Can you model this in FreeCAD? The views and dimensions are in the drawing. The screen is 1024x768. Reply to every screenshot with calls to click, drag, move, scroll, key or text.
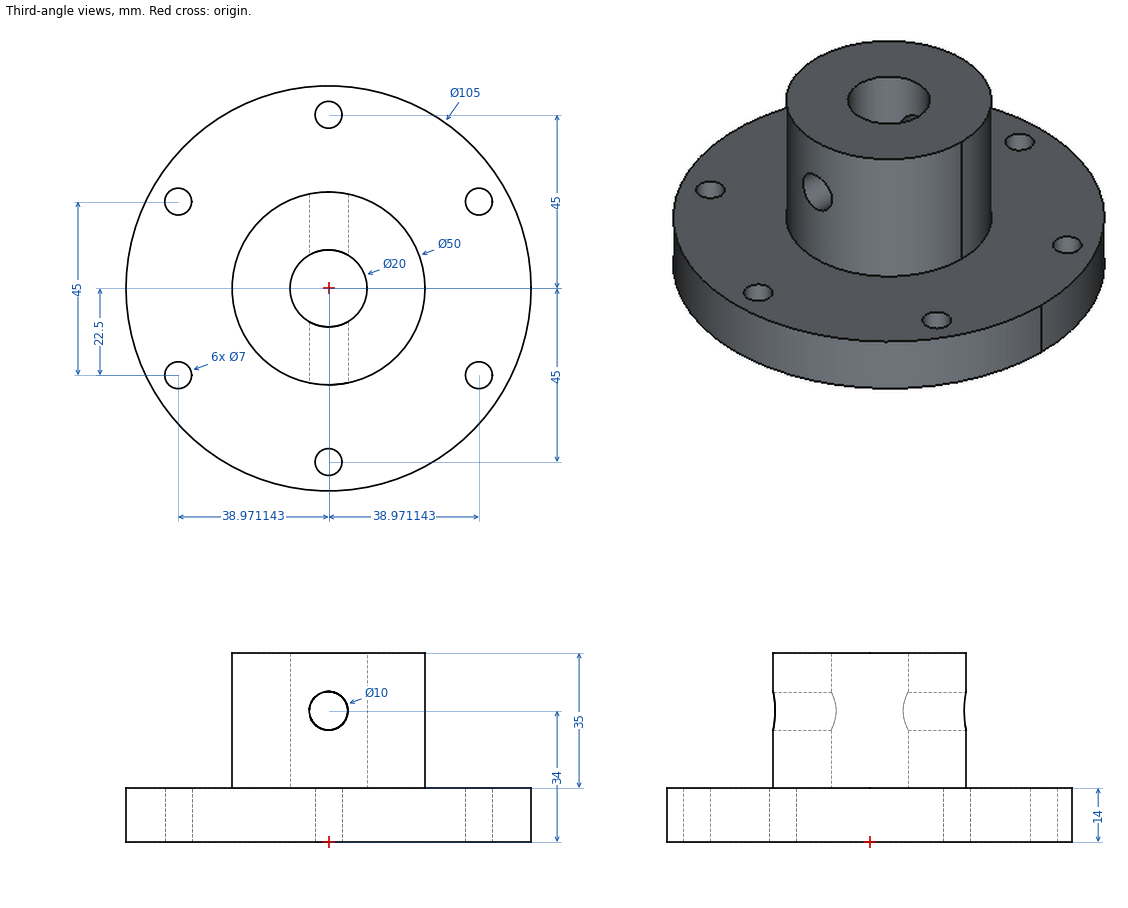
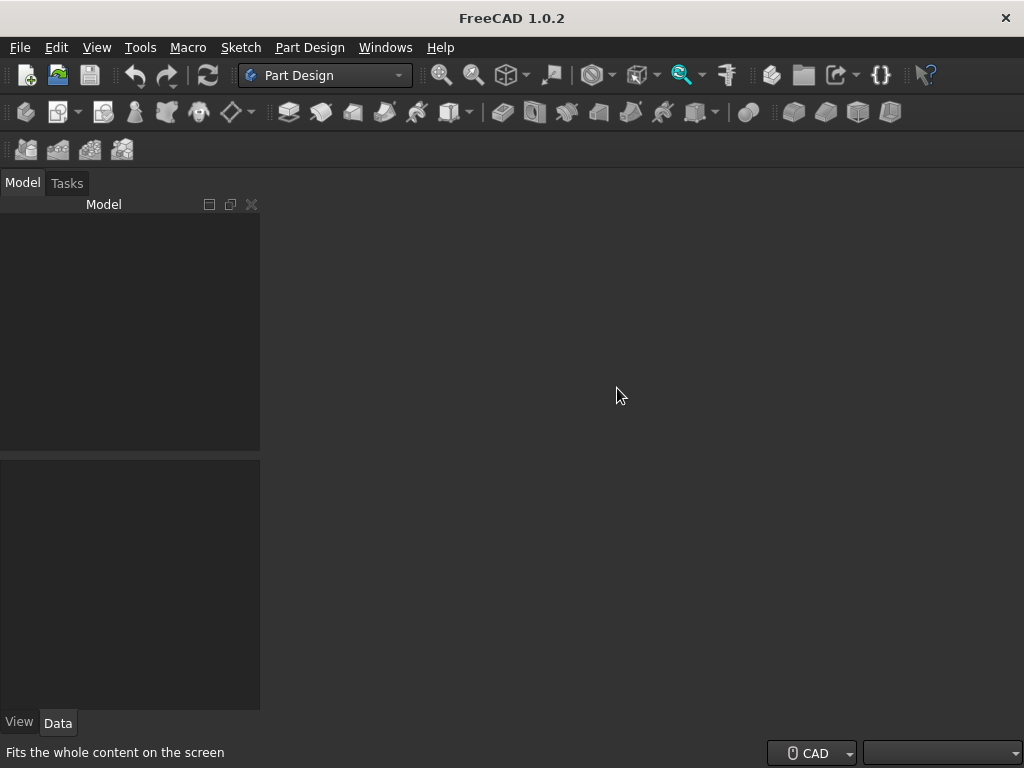
click(26, 76)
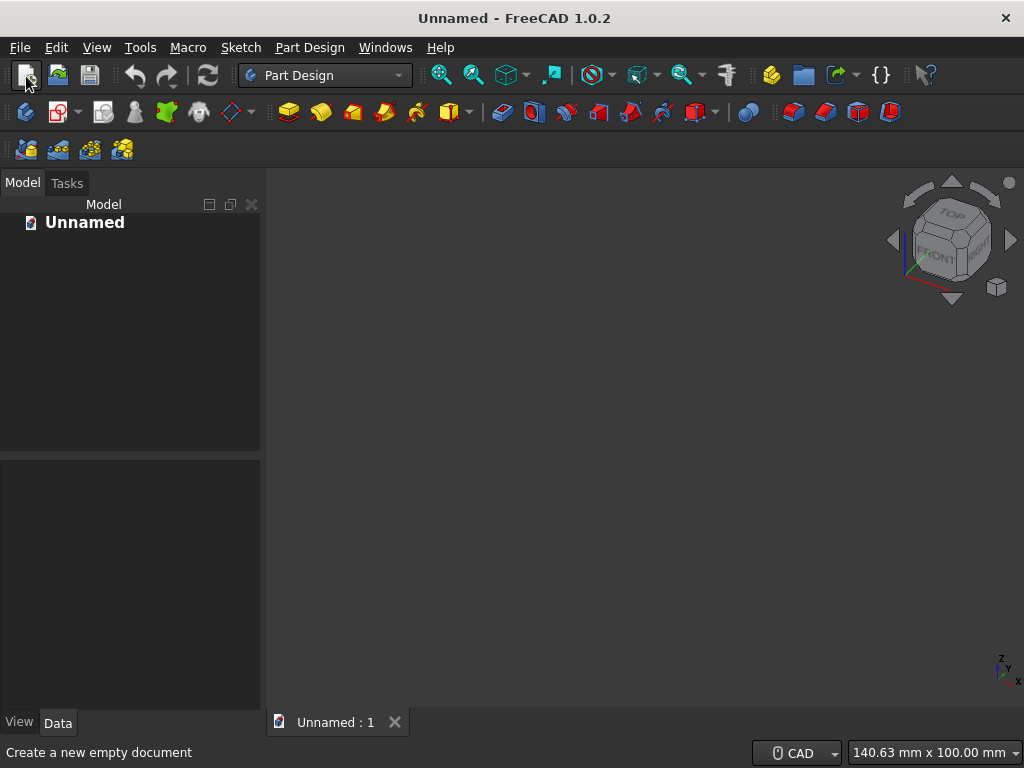
click(58, 112)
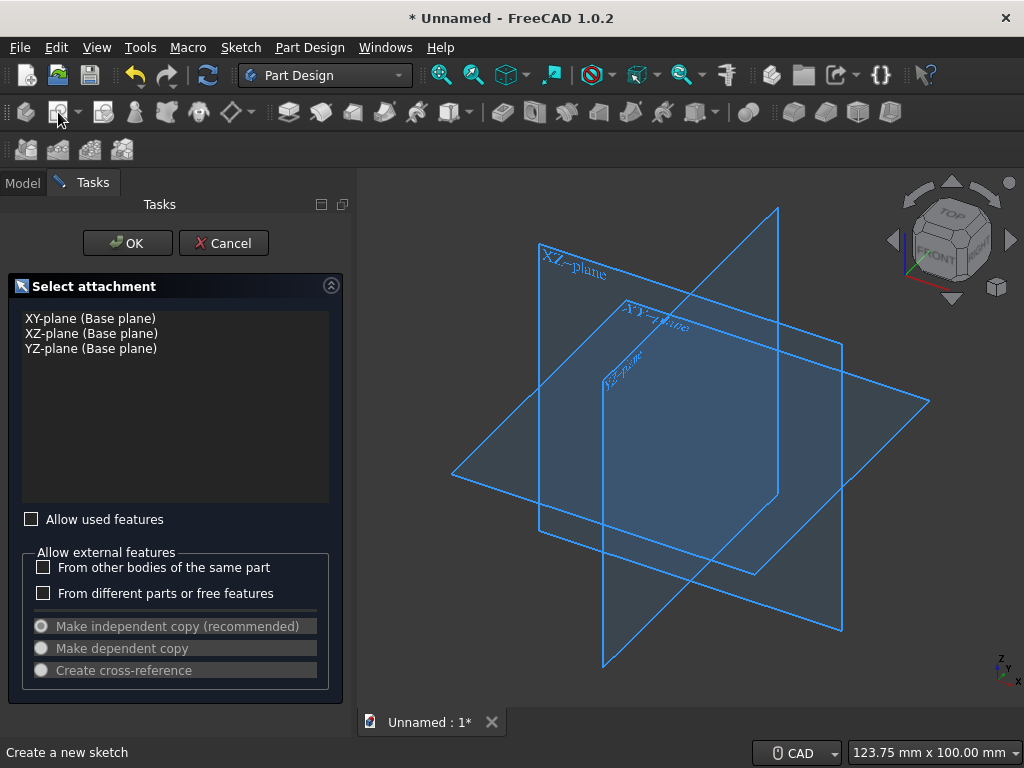
click(82, 318)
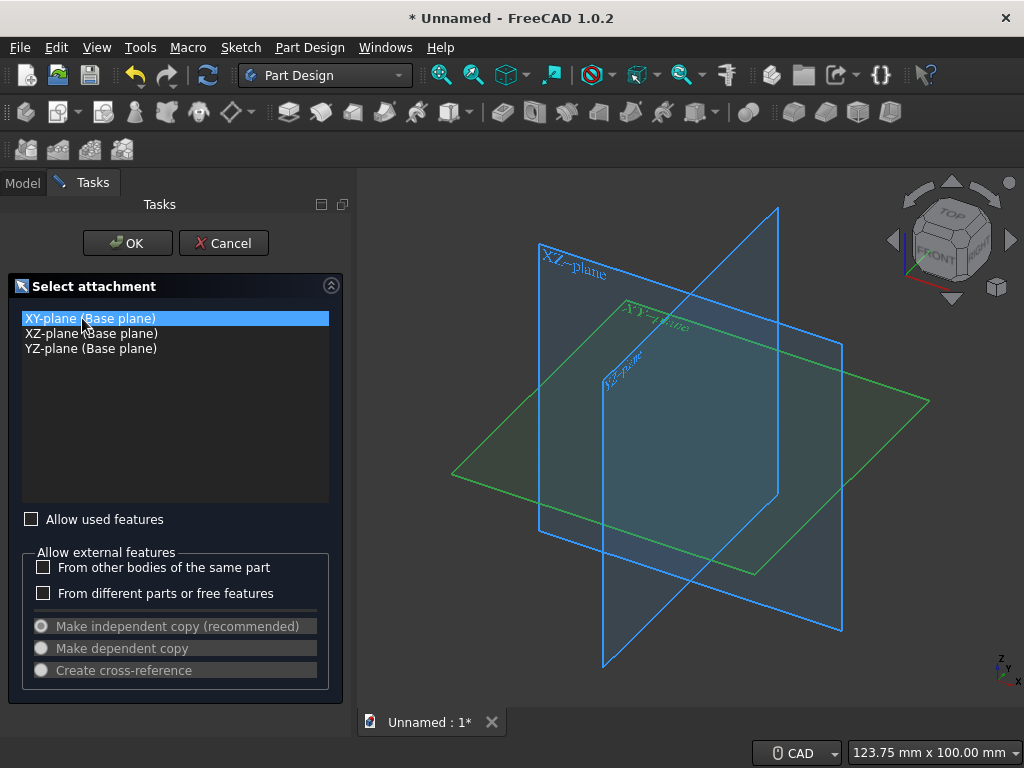
click(128, 243)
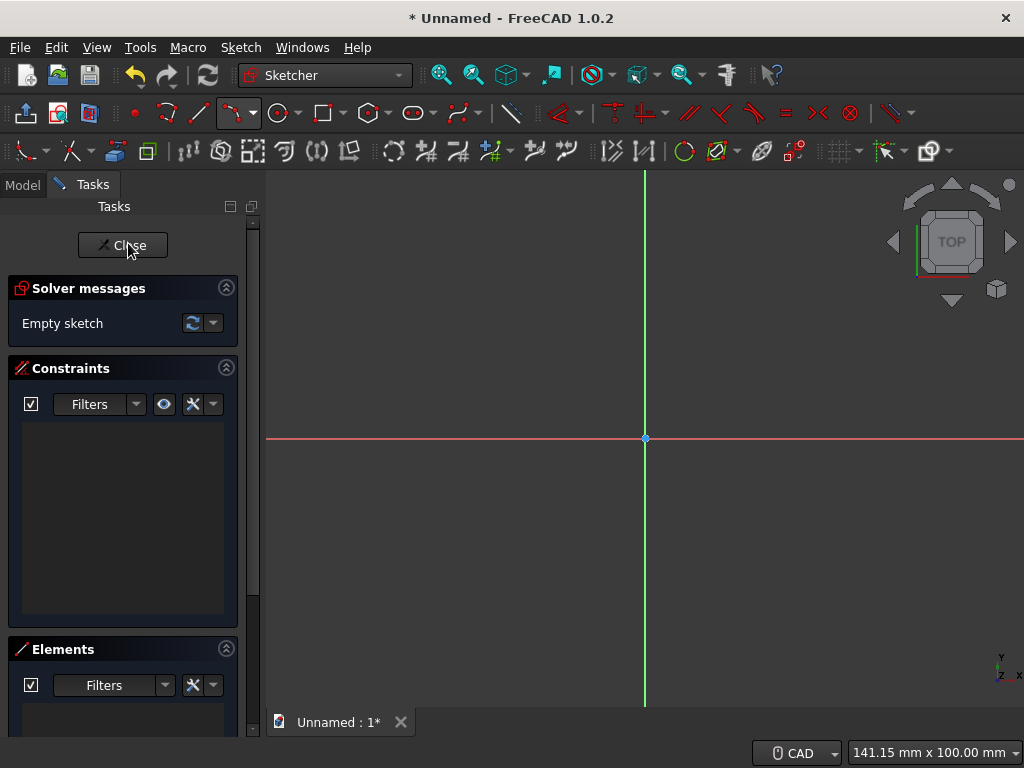
scroll(493, 438, down, 3)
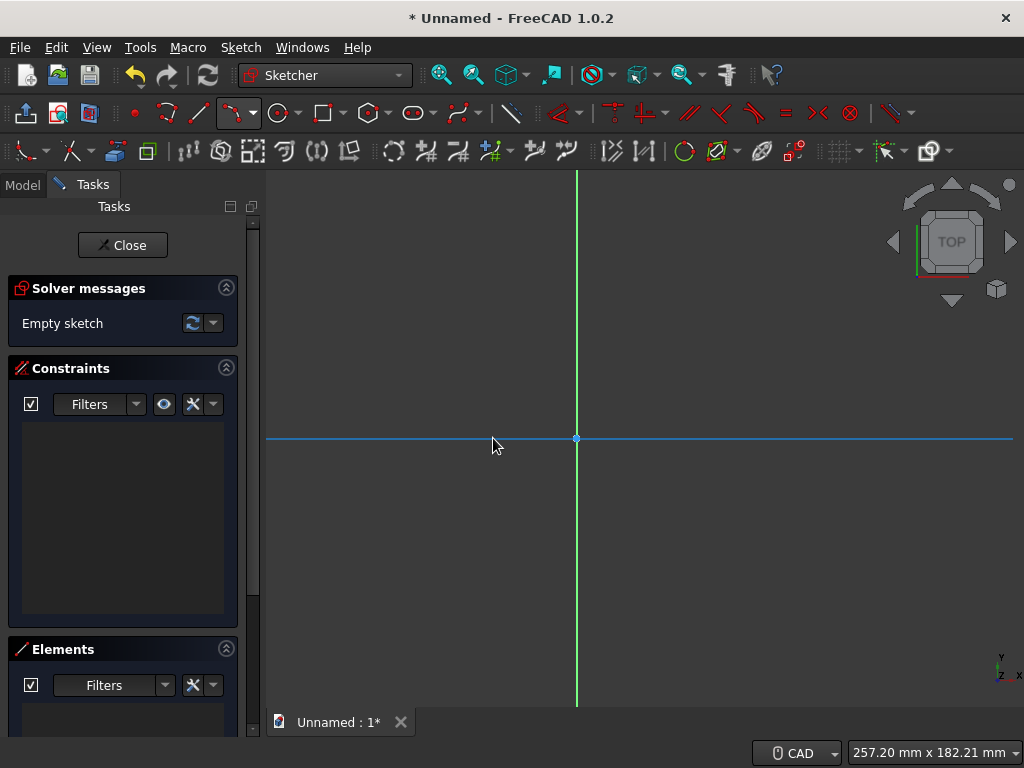
key(g)
key(c)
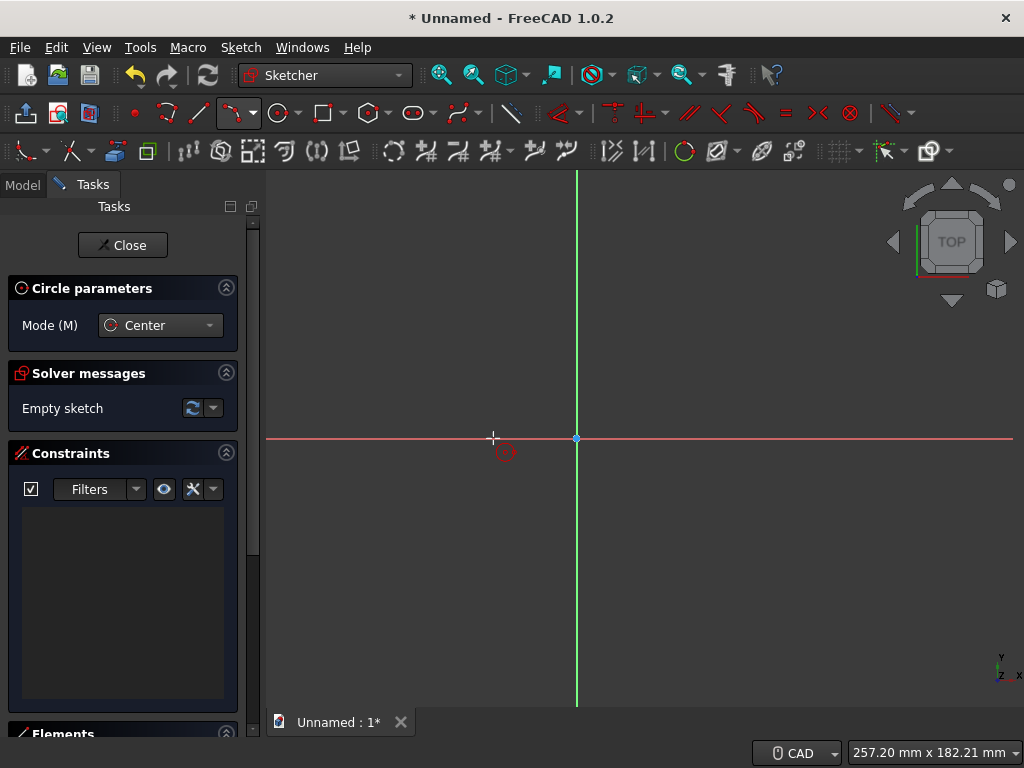
click(577, 438)
move(686, 329)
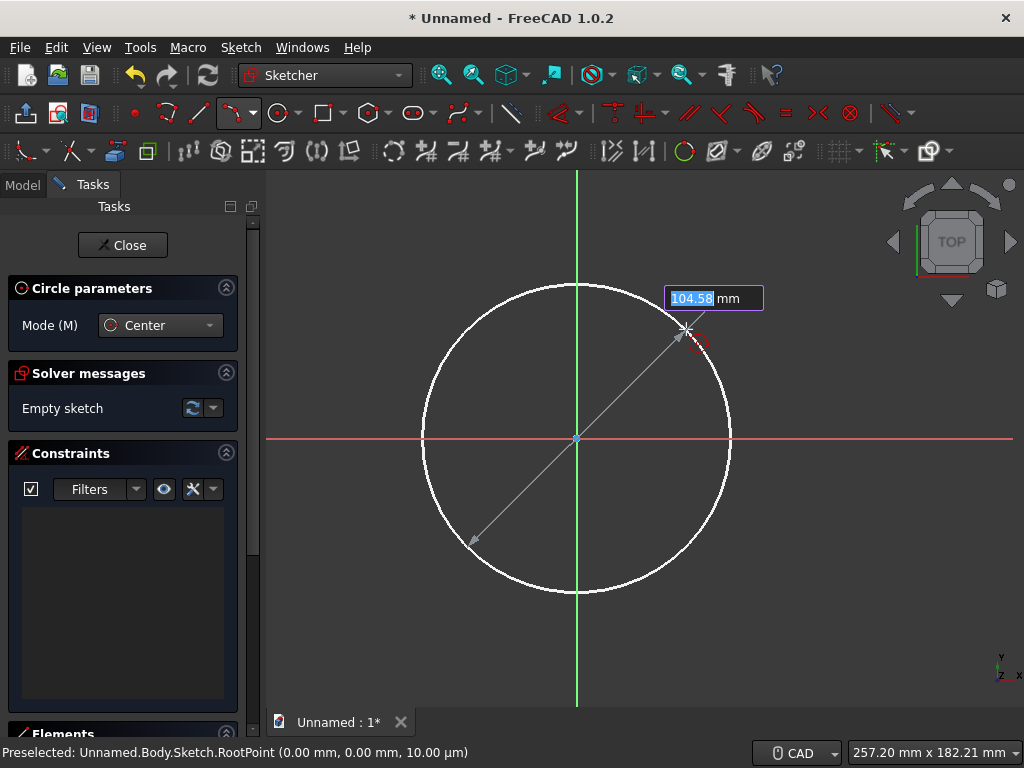
text(105)
key(Return)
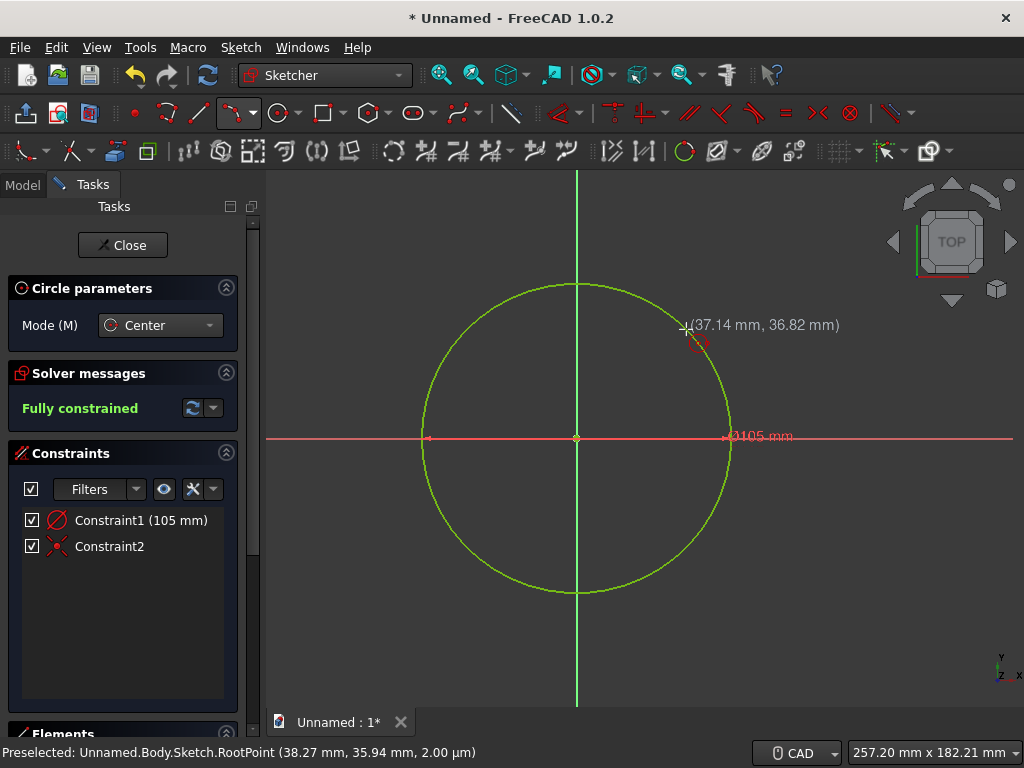
scroll(462, 505, up, 4)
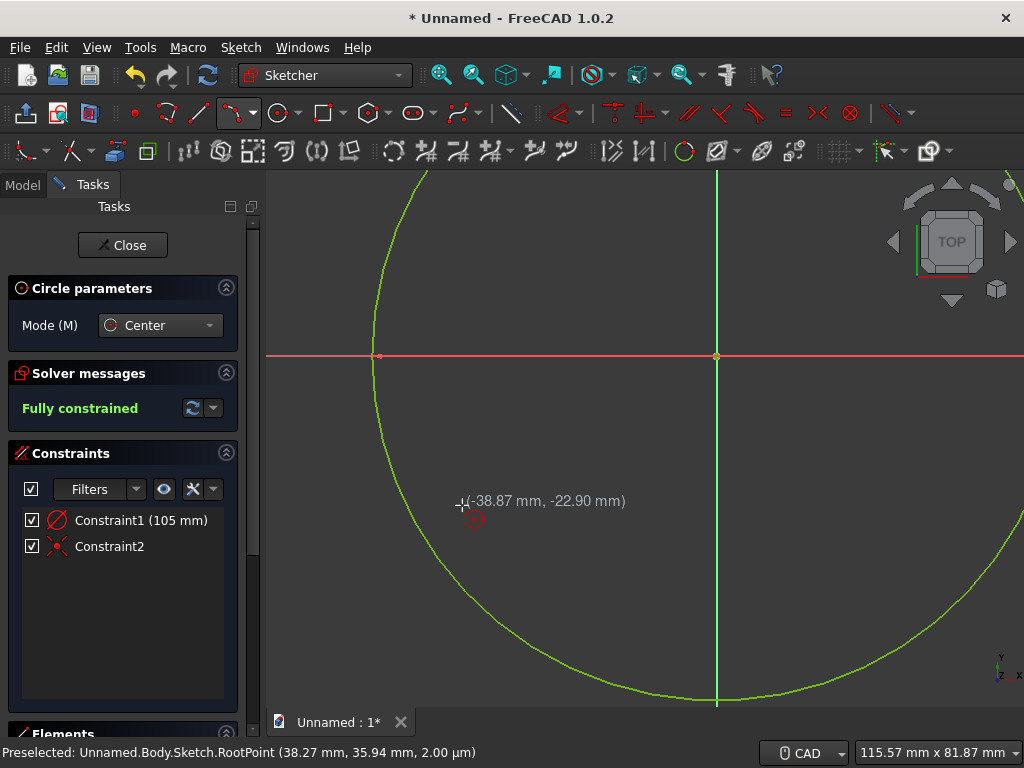
click(461, 504)
move(477, 488)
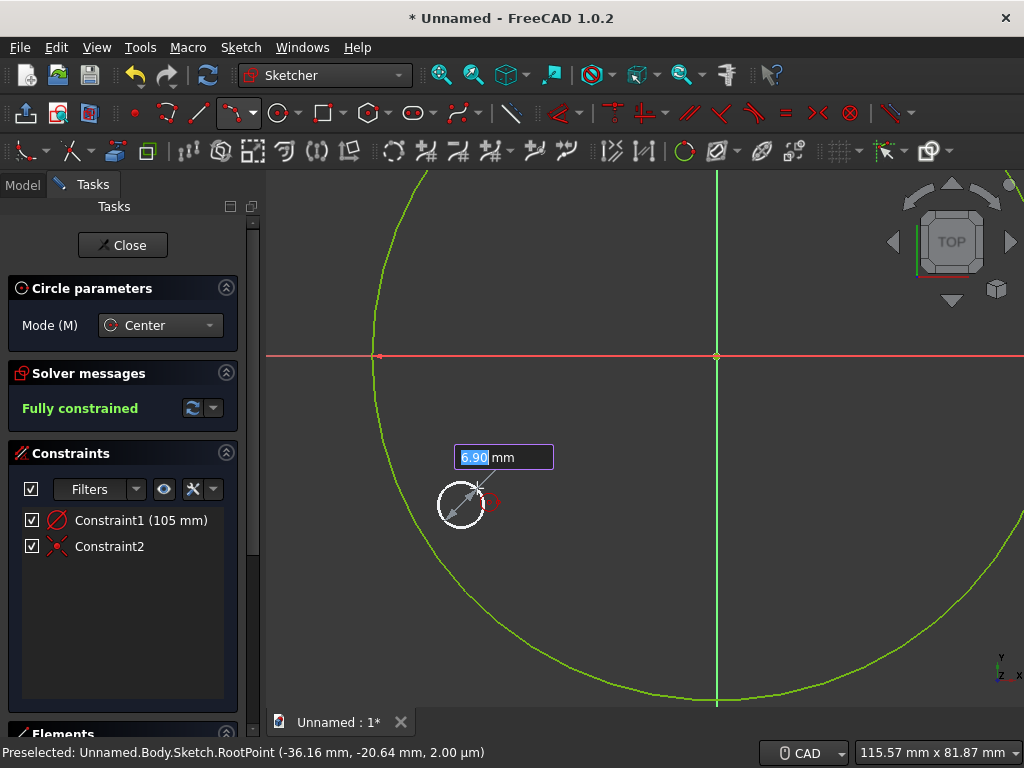
text(7)
key(Return)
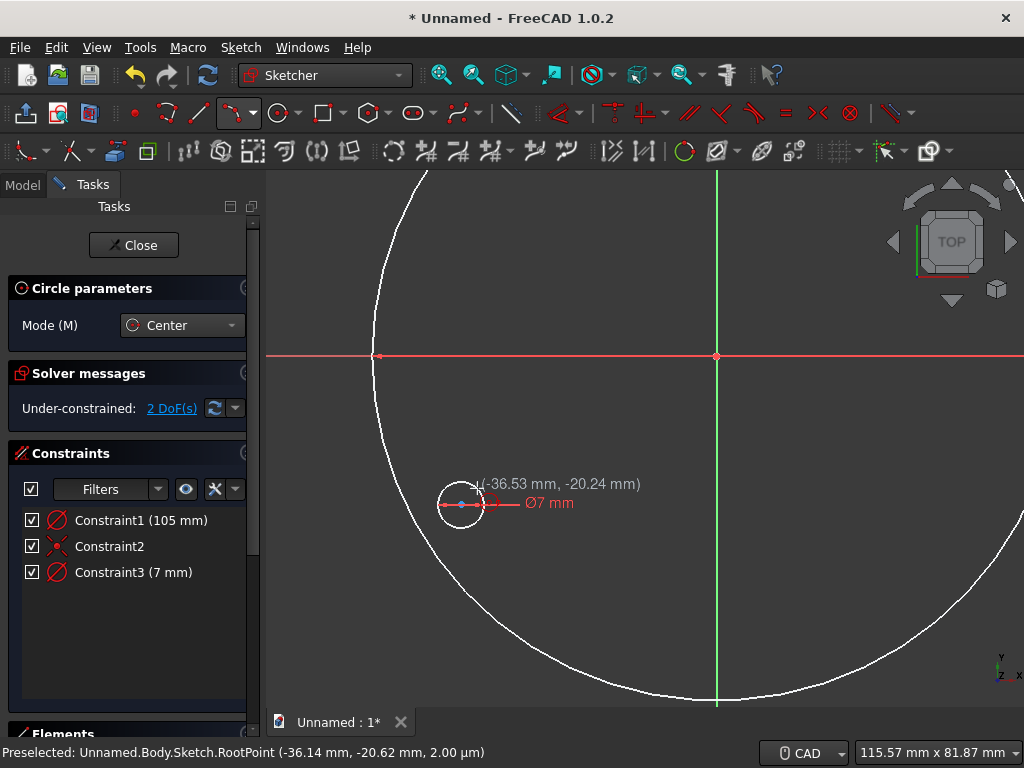
click(717, 651)
move(733, 635)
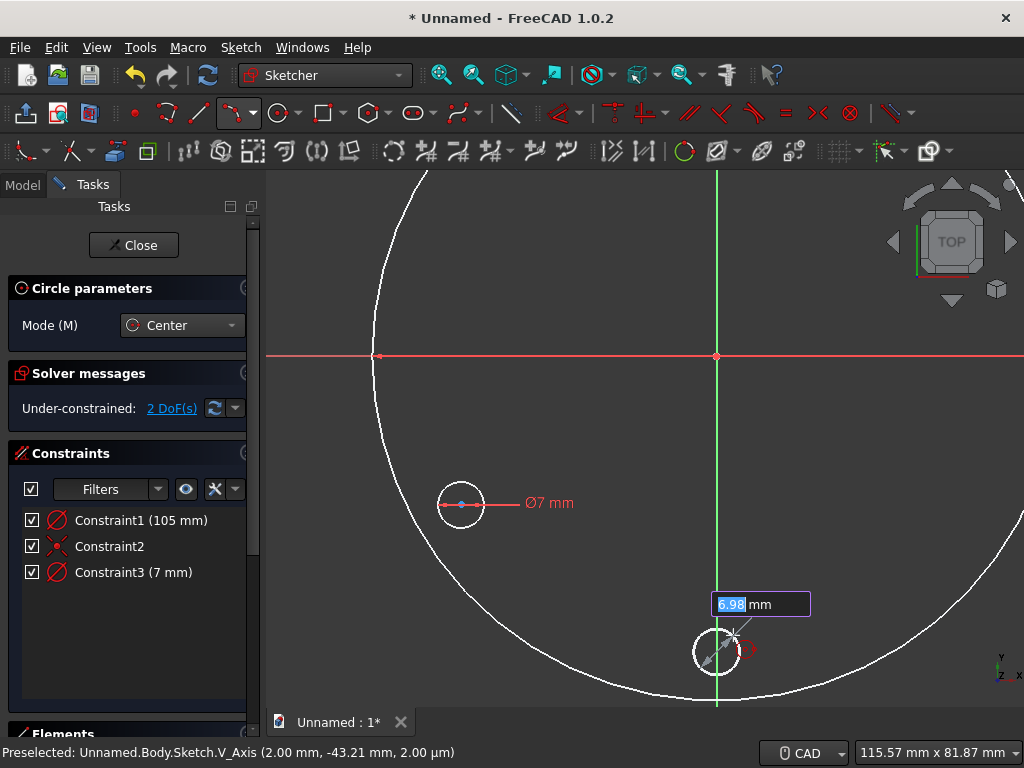
text(7)
key(Return)